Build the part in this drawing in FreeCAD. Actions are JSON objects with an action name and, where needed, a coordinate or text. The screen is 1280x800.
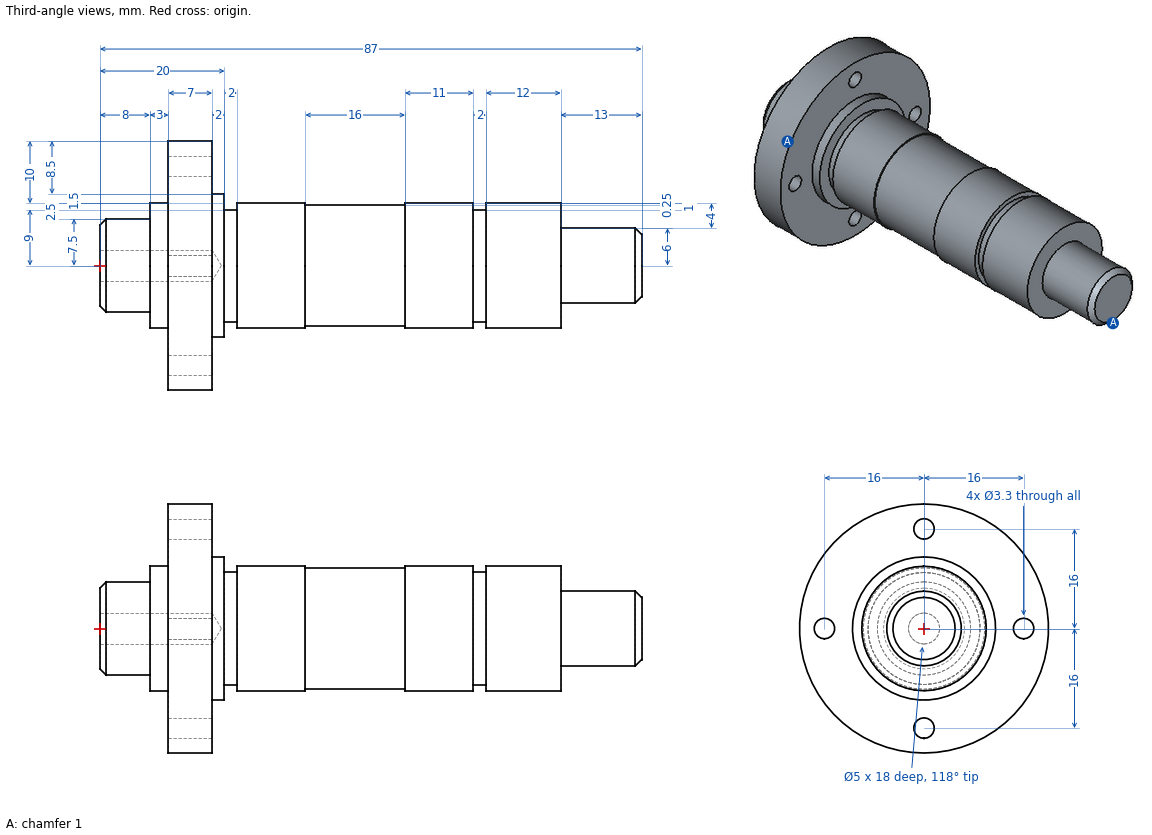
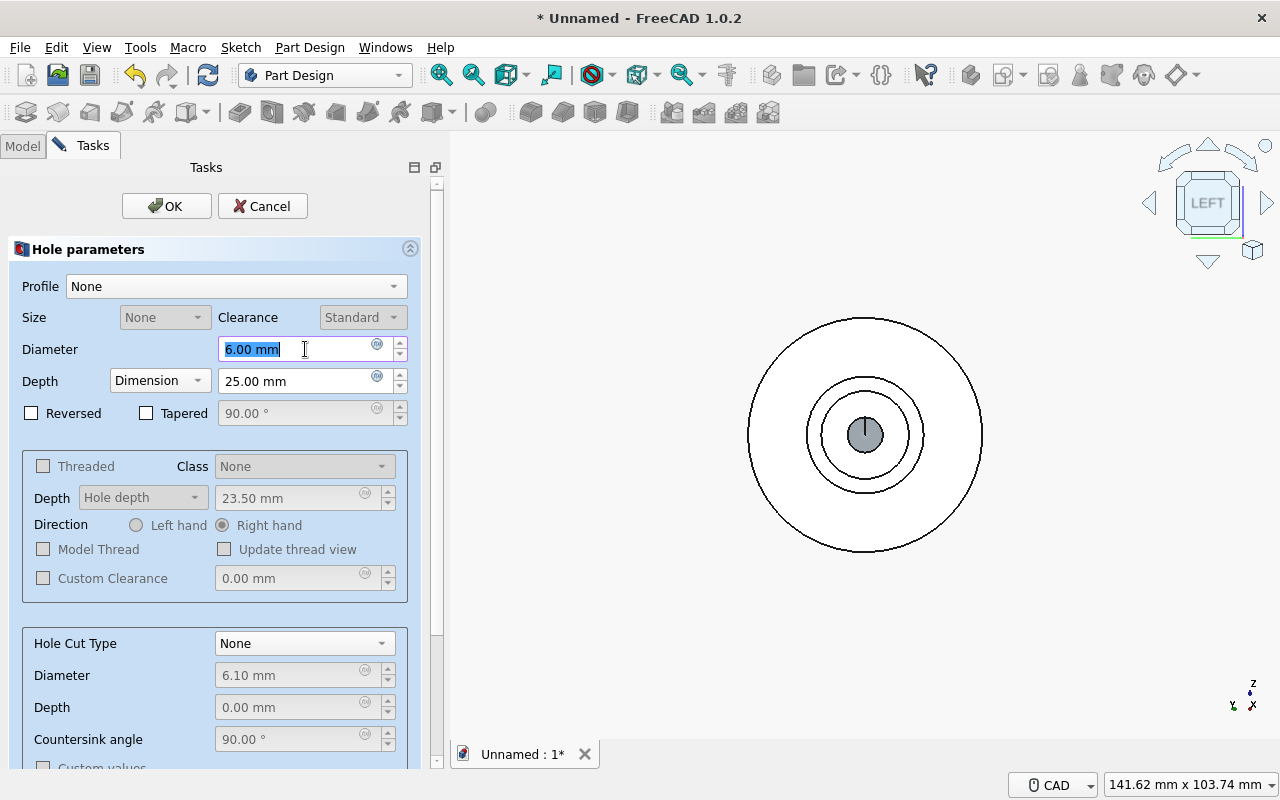
{"action": "type", "text": "5"}
{"action": "key", "text": "Tab"}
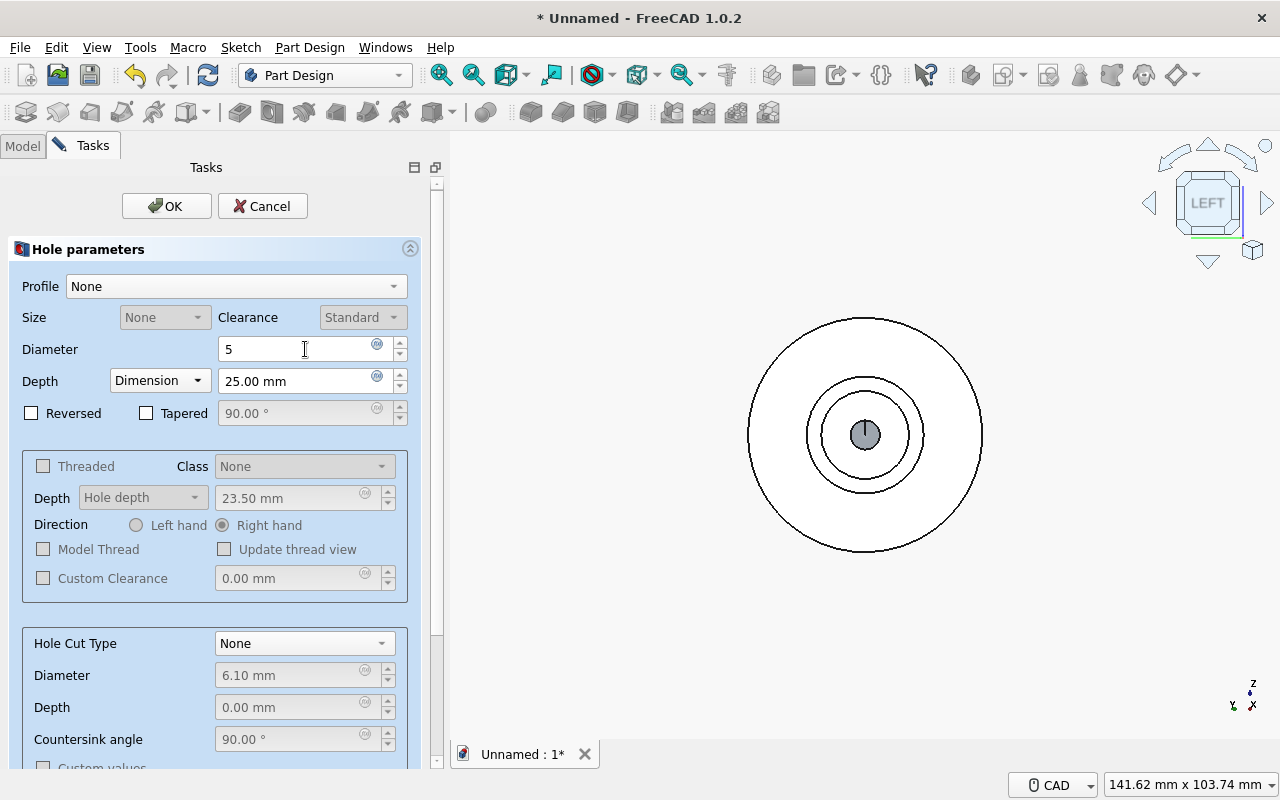
{"action": "triple_click", "coordinate": [305, 381]}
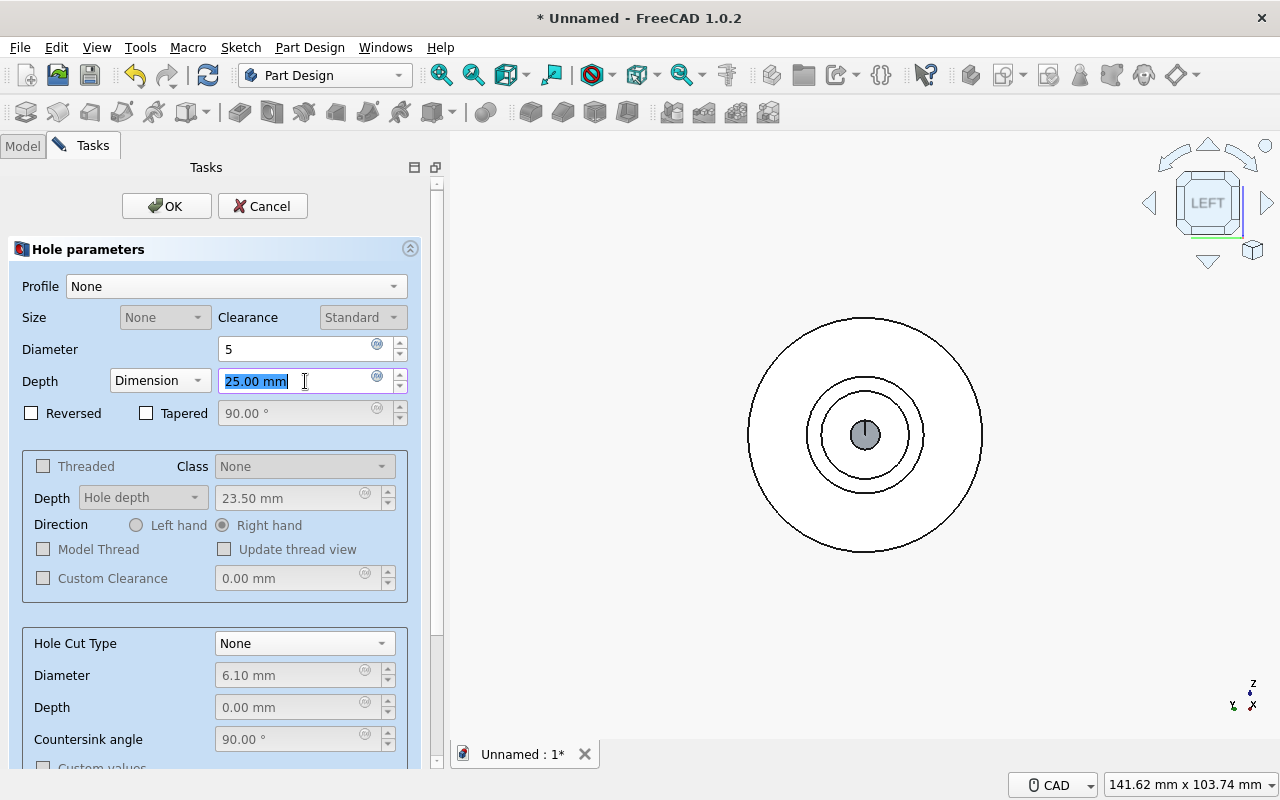
{"action": "type", "text": "18"}
{"action": "key", "text": "Tab"}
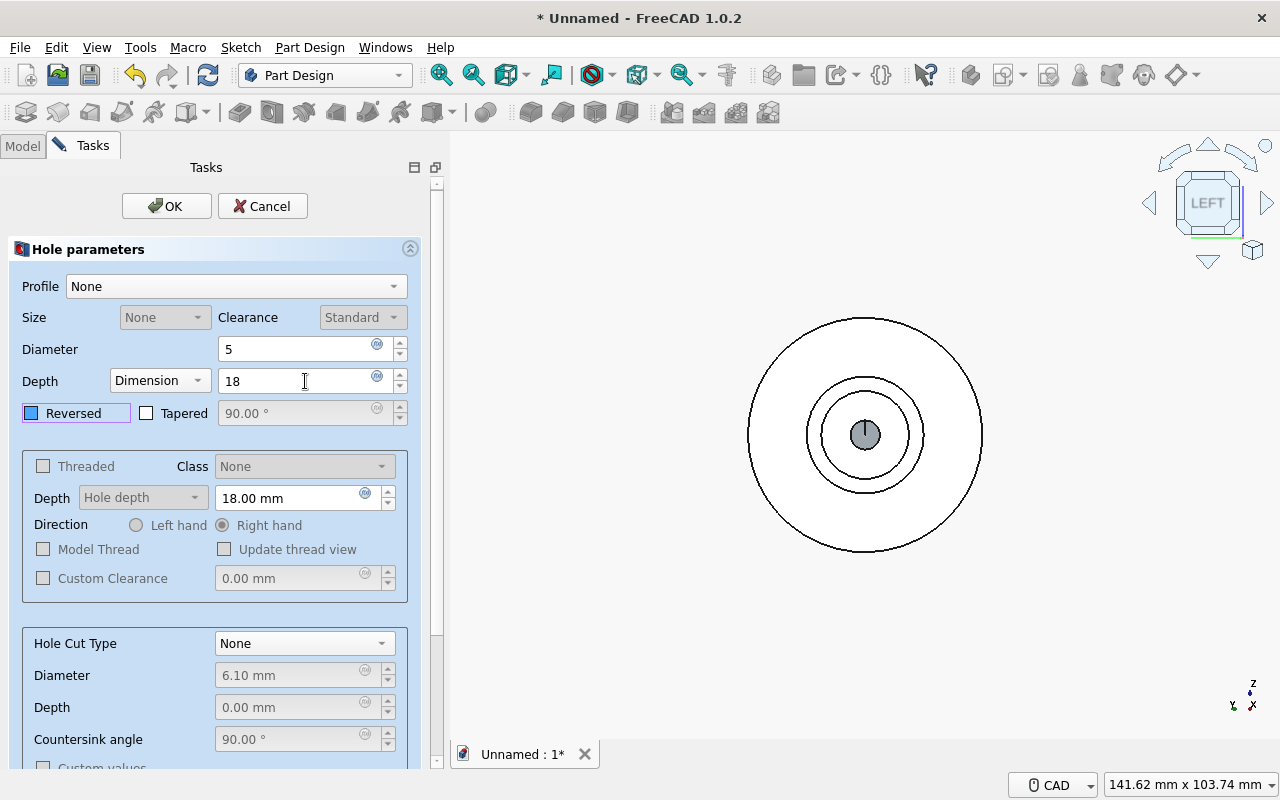
{"action": "left_click", "coordinate": [167, 206]}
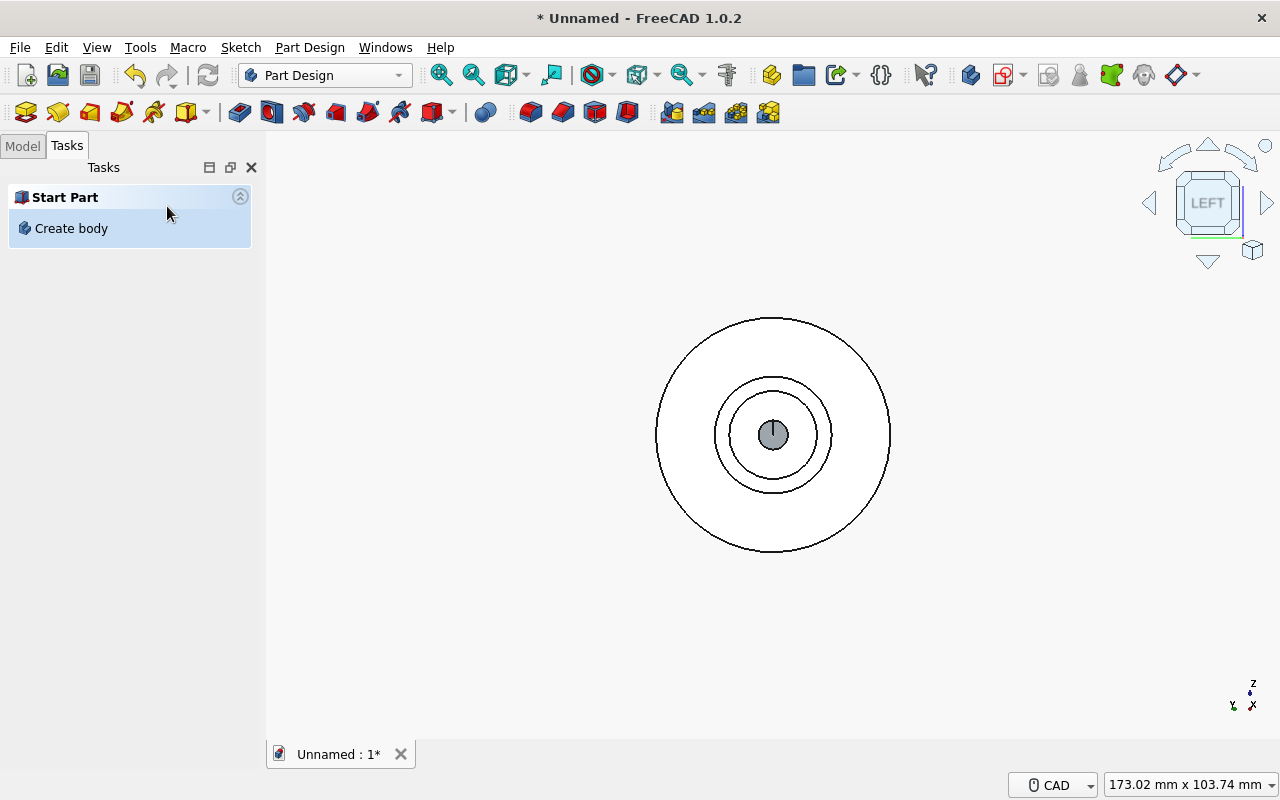
{"action": "left_click", "coordinate": [442, 76]}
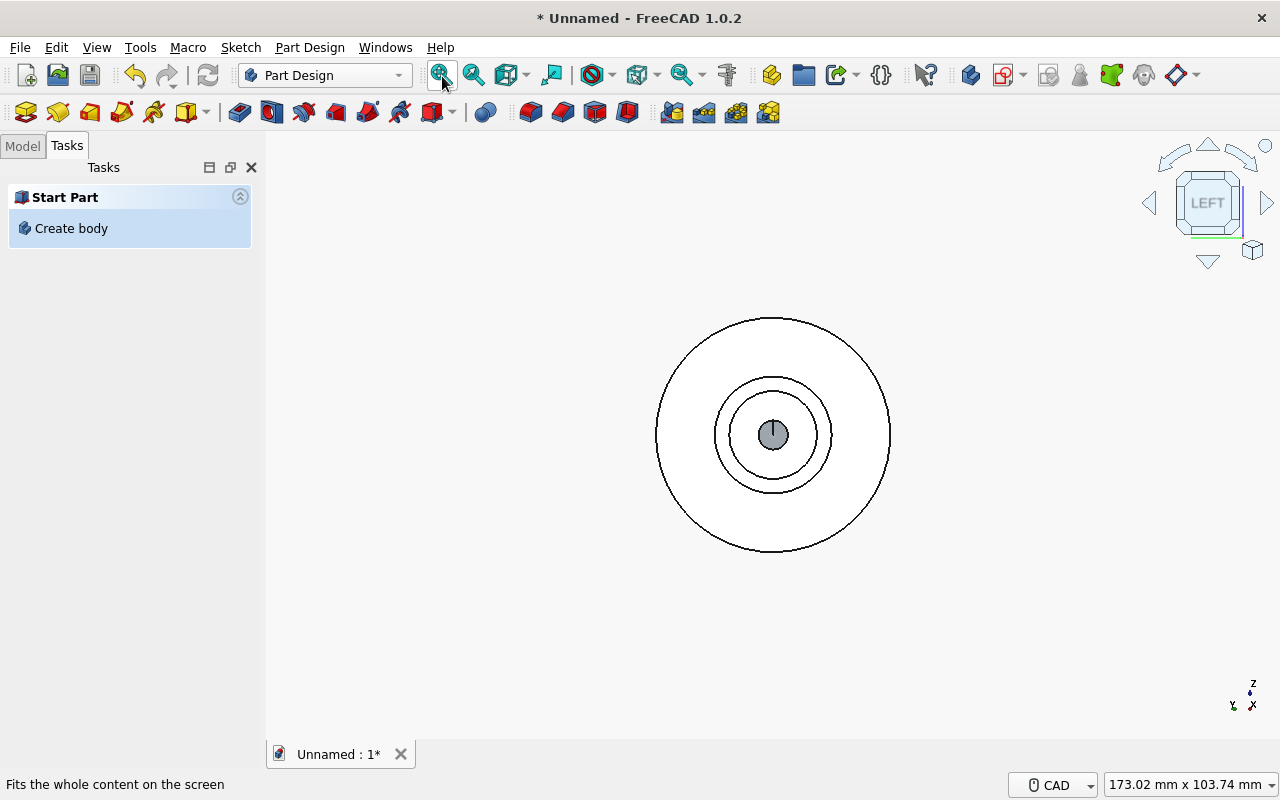
{"action": "left_click", "coordinate": [706, 367]}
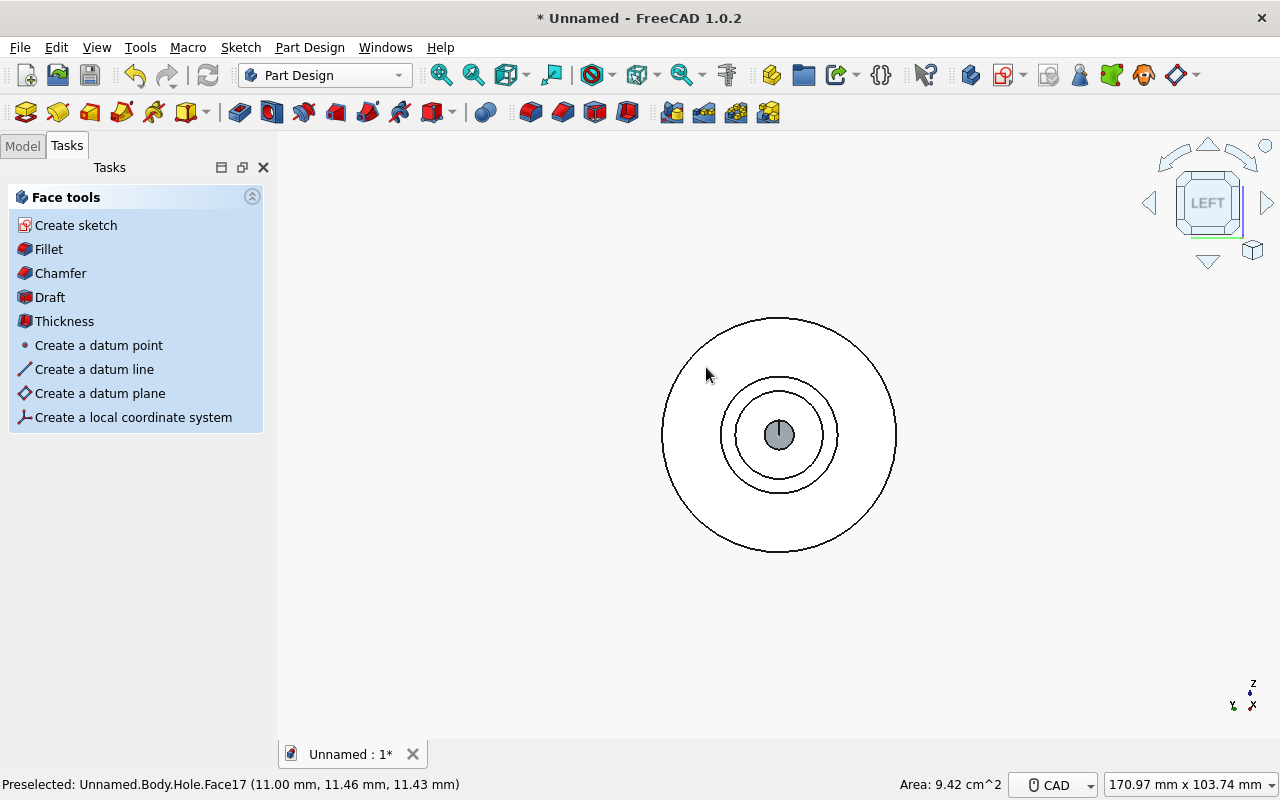
{"action": "left_click", "coordinate": [1004, 76]}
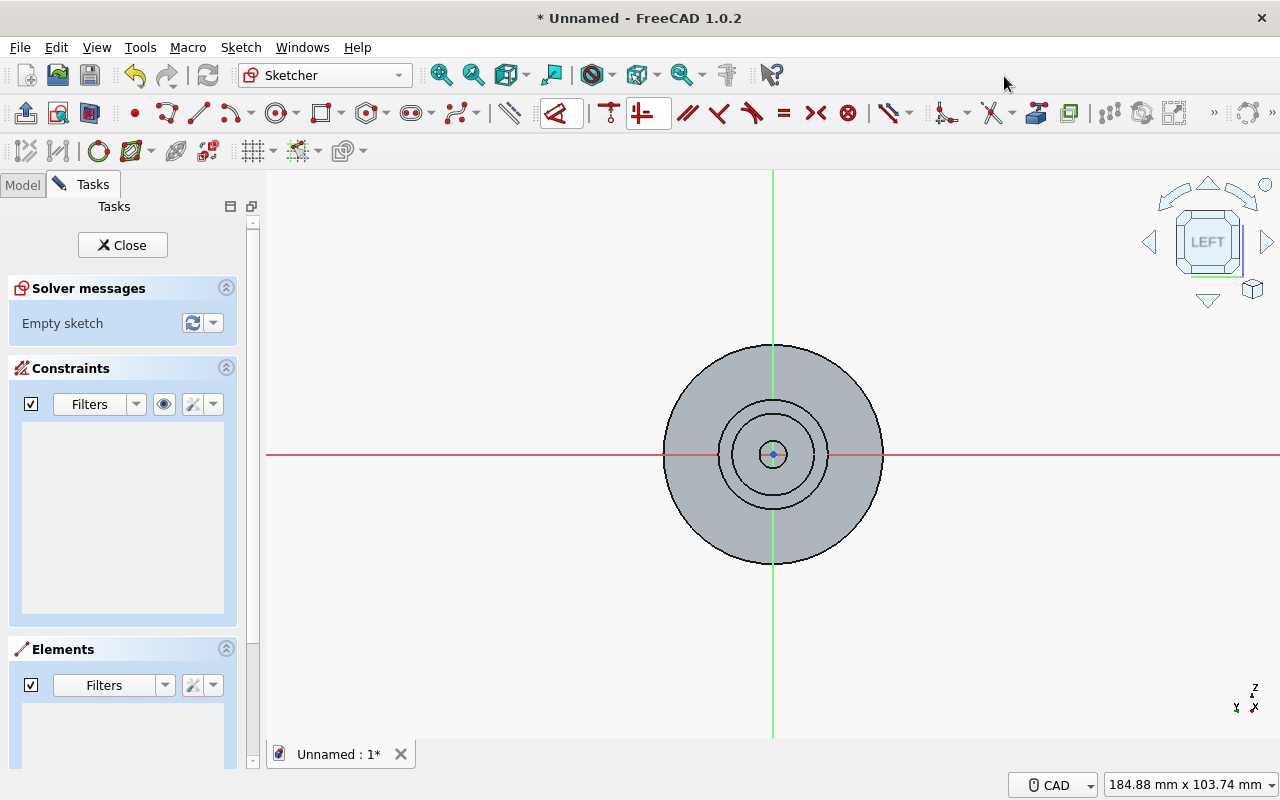
{"action": "left_click", "coordinate": [90, 114]}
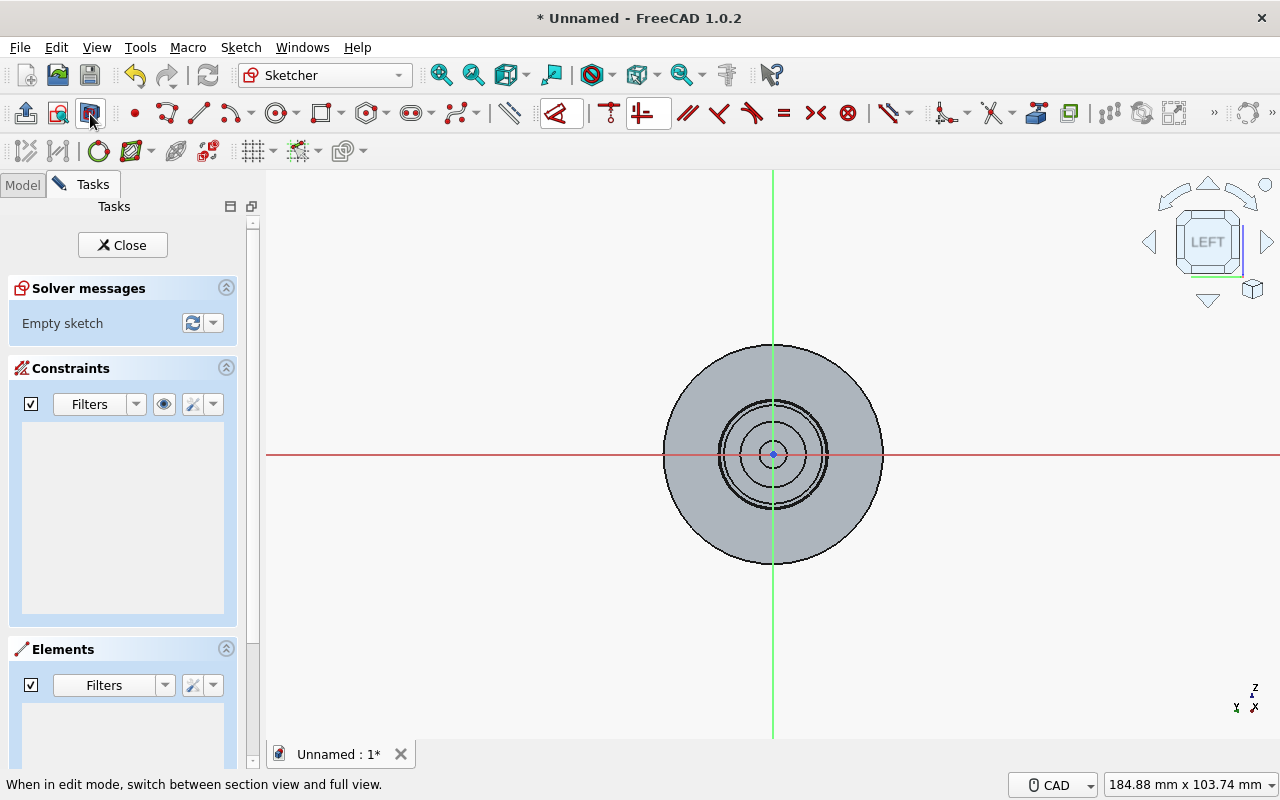
{"action": "scroll", "coordinate": [857, 454], "scroll_direction": "up", "scroll_amount": 3}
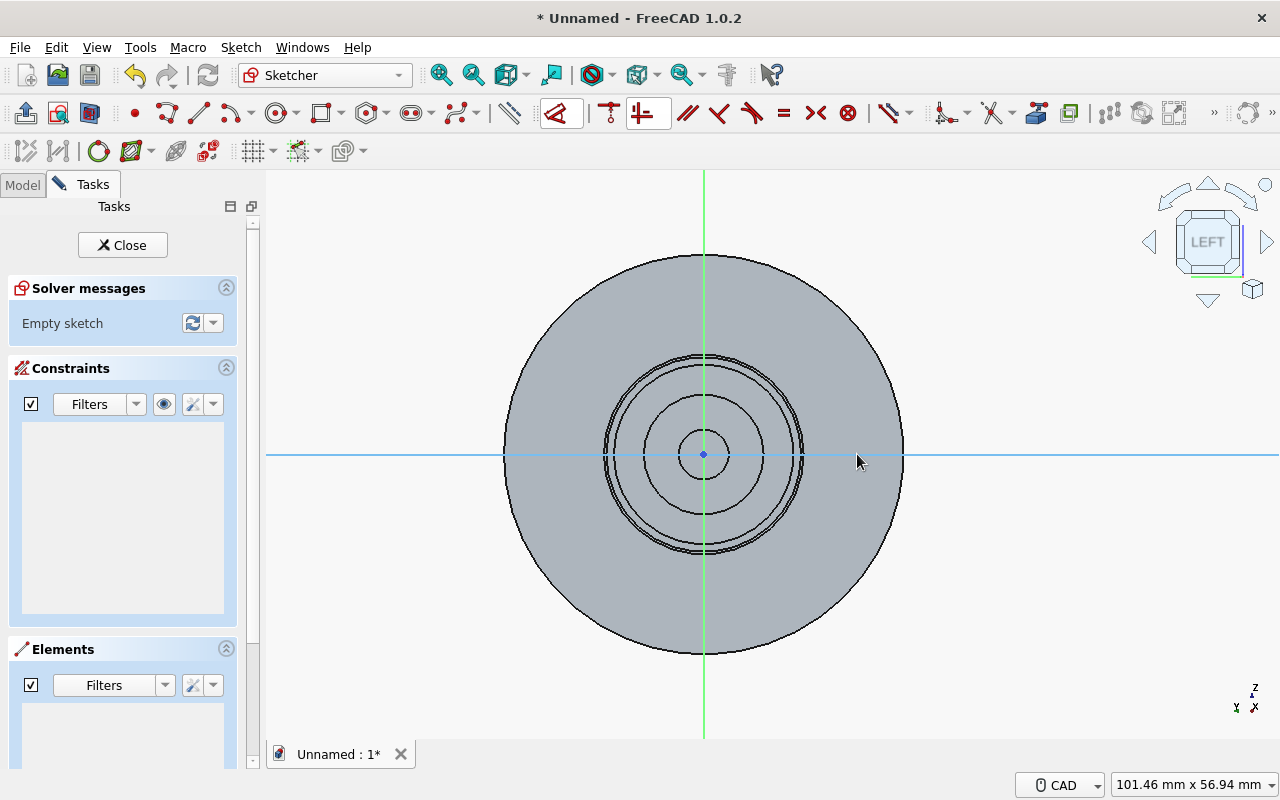
{"action": "left_click", "coordinate": [276, 114]}